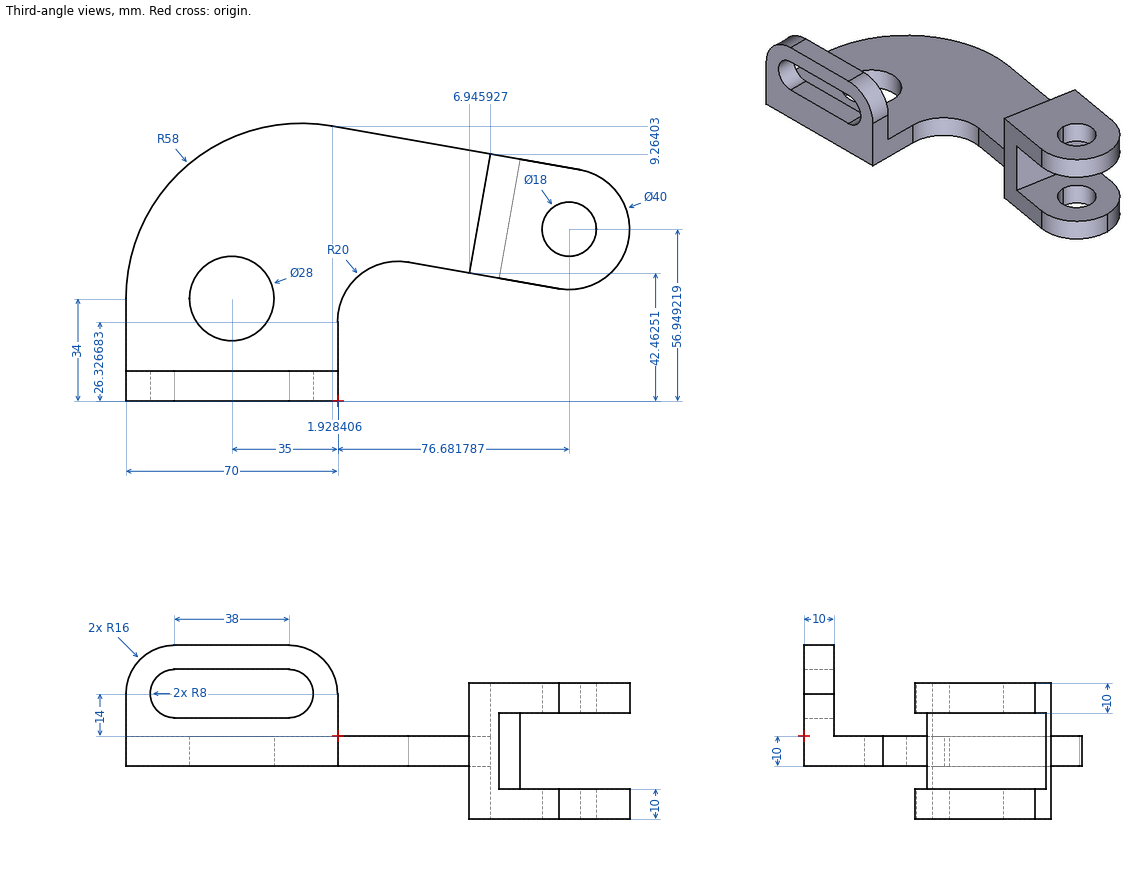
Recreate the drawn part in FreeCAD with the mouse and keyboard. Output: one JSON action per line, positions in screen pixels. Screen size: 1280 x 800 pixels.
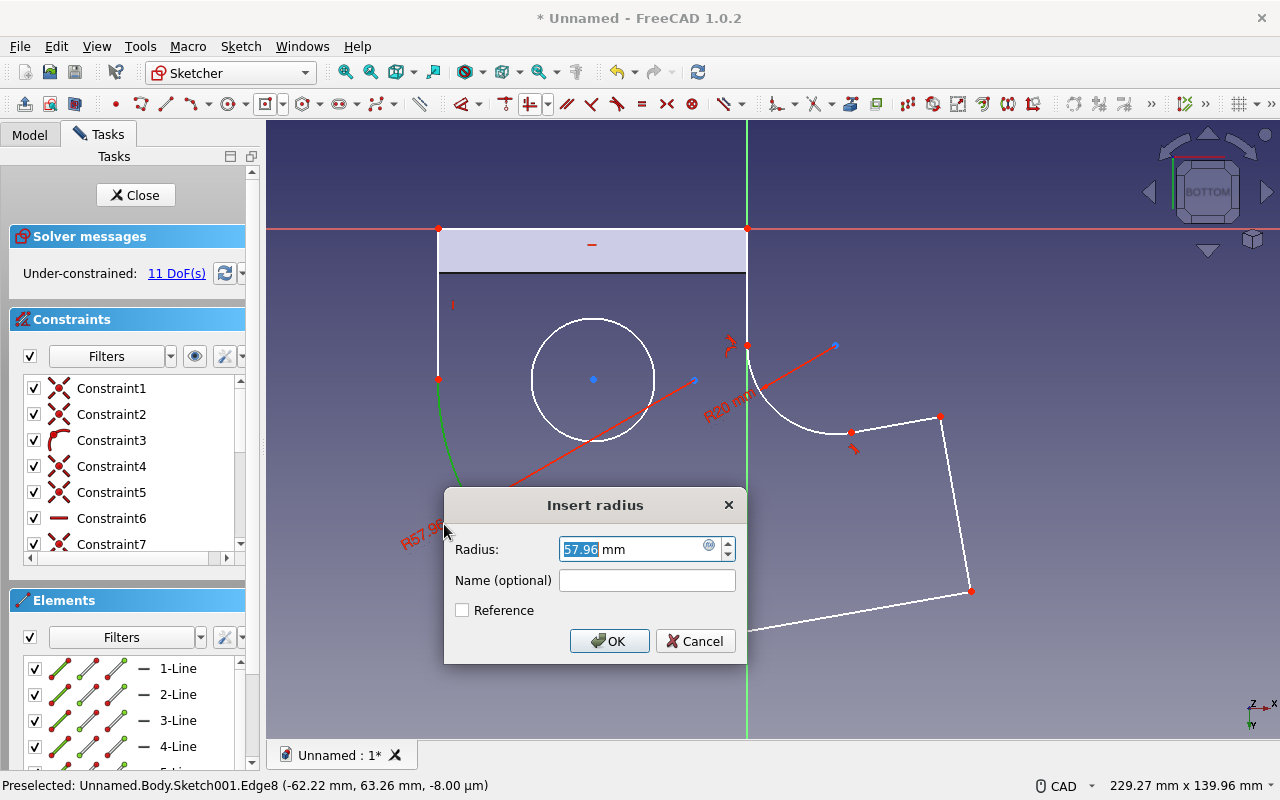
{"action": "type", "text": "58"}
{"action": "key", "text": "Return"}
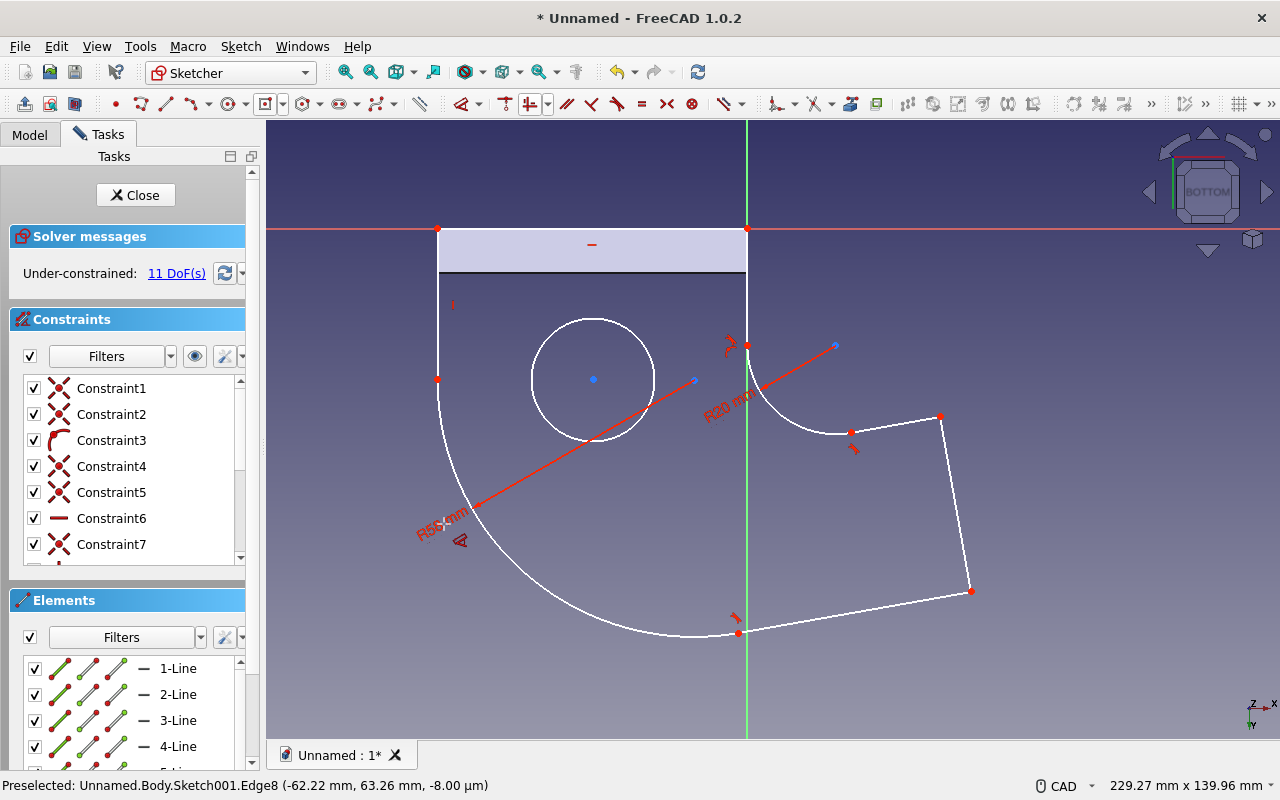
{"action": "left_click", "coordinate": [636, 336]}
{"action": "left_click", "coordinate": [658, 313]}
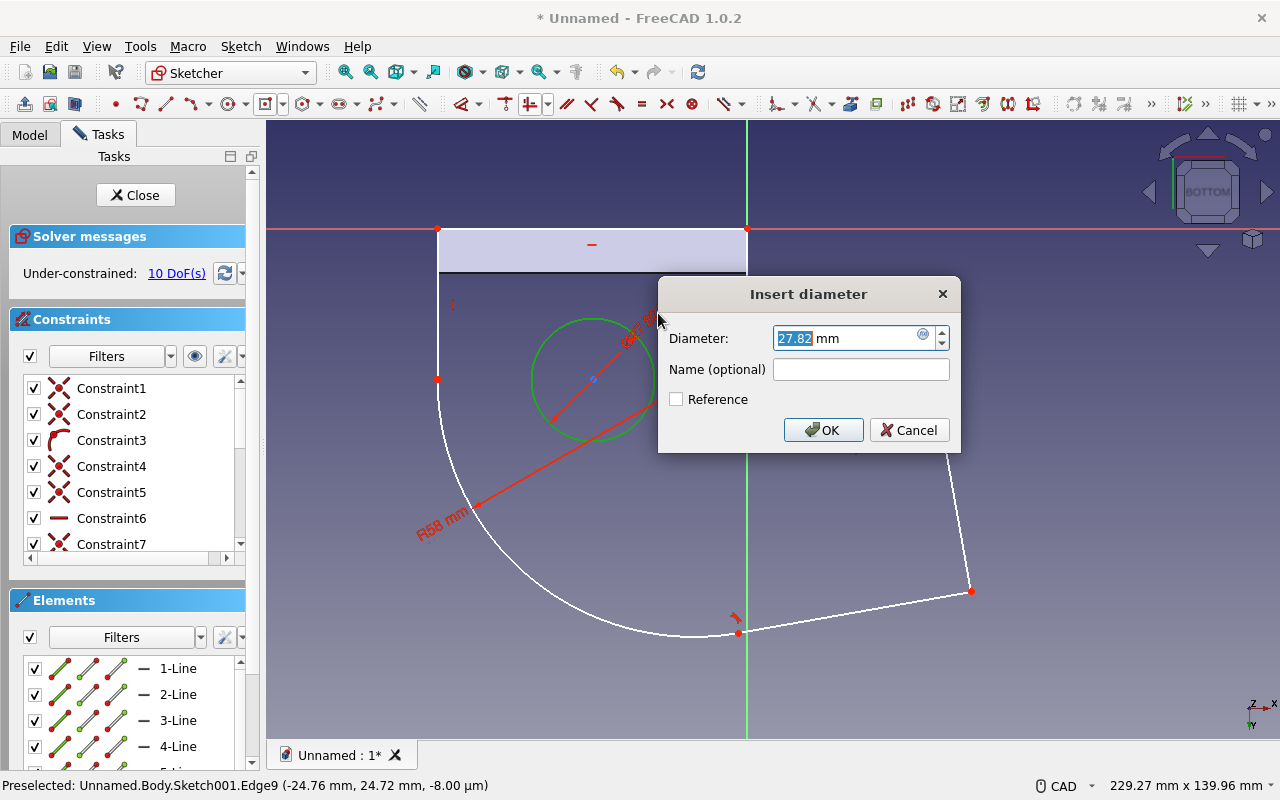
{"action": "type", "text": "28"}
{"action": "key", "text": "Return"}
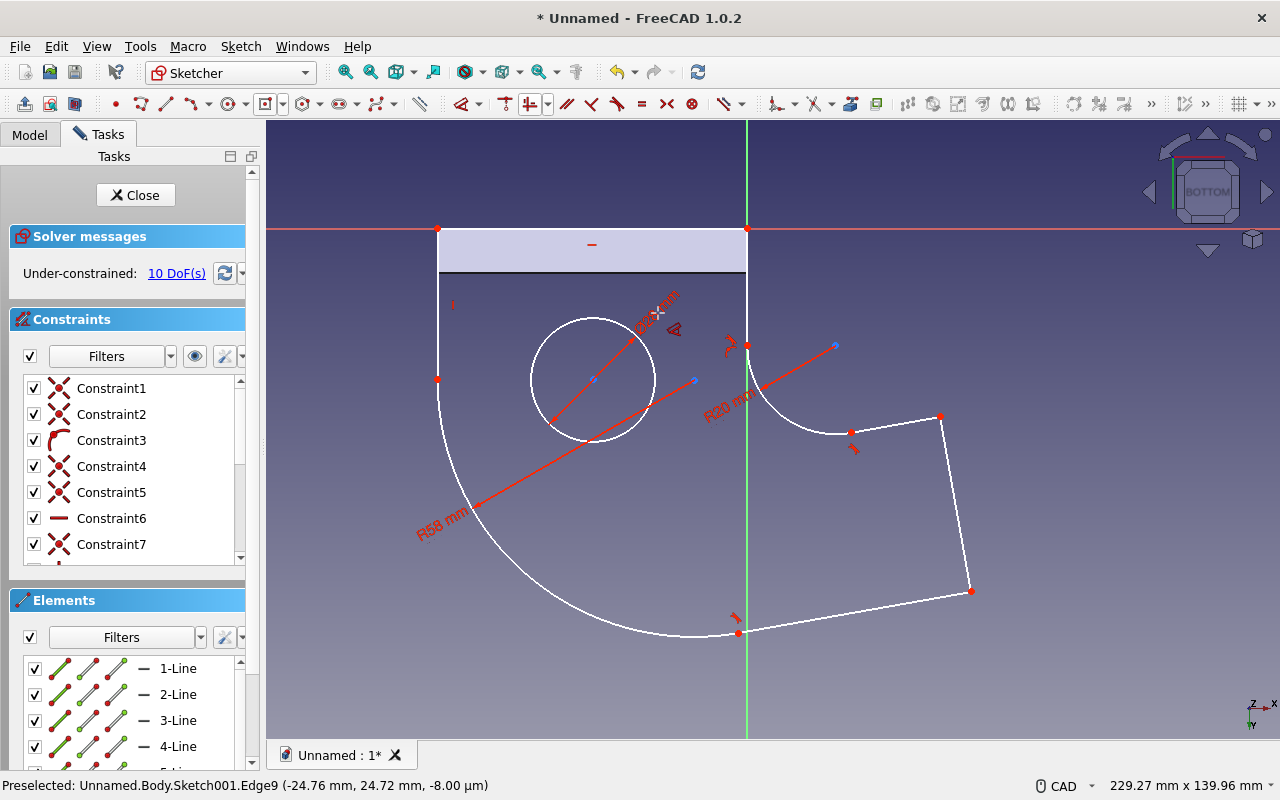
{"action": "left_click", "coordinate": [654, 229]}
{"action": "left_click", "coordinate": [593, 195]}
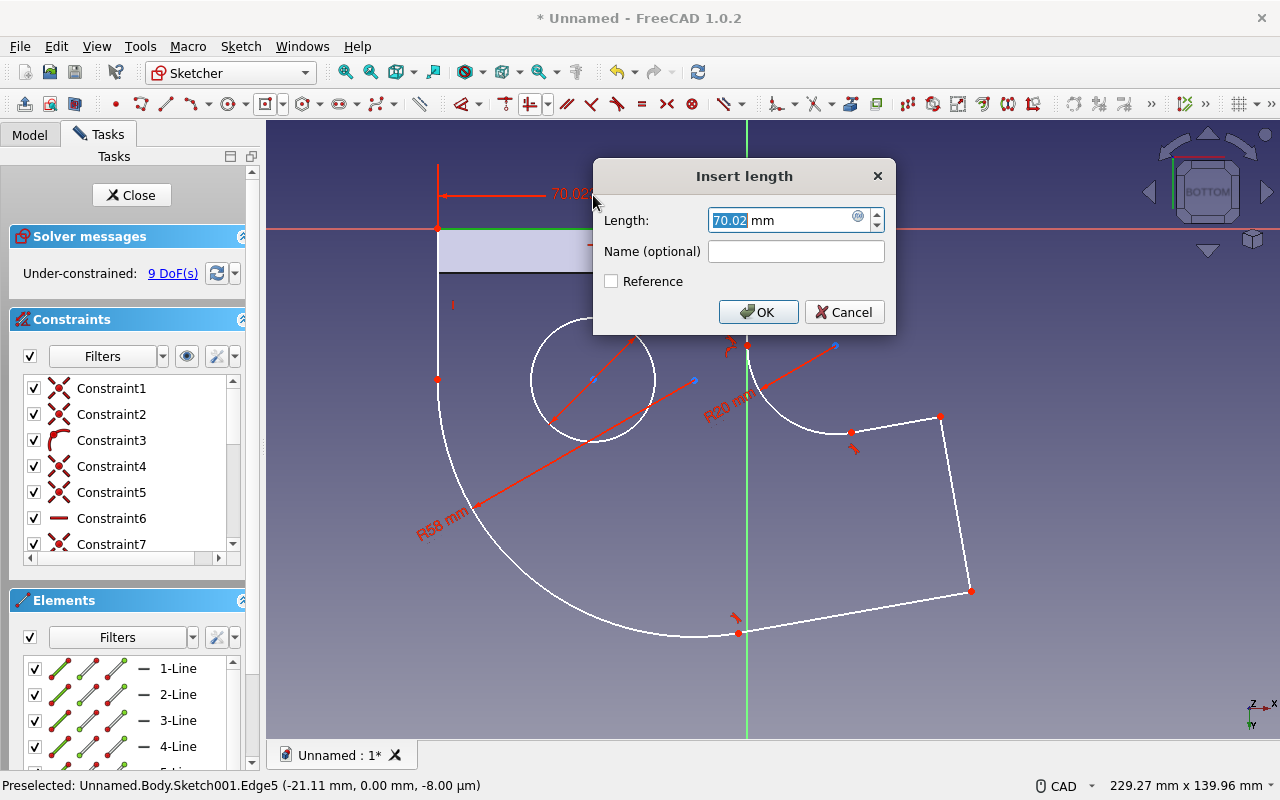
{"action": "type", "text": "70"}
{"action": "key", "text": "Return"}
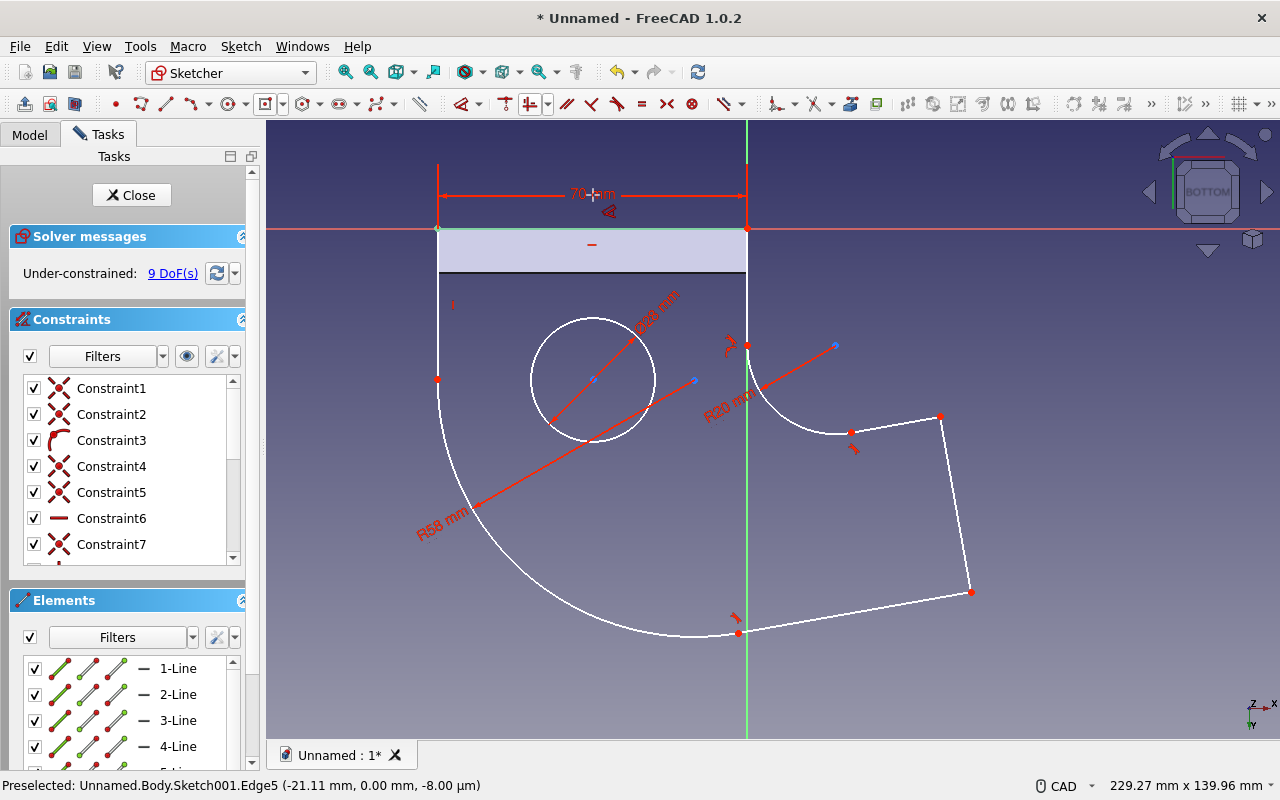
{"action": "left_click", "coordinate": [438, 274]}
{"action": "left_click", "coordinate": [404, 304]}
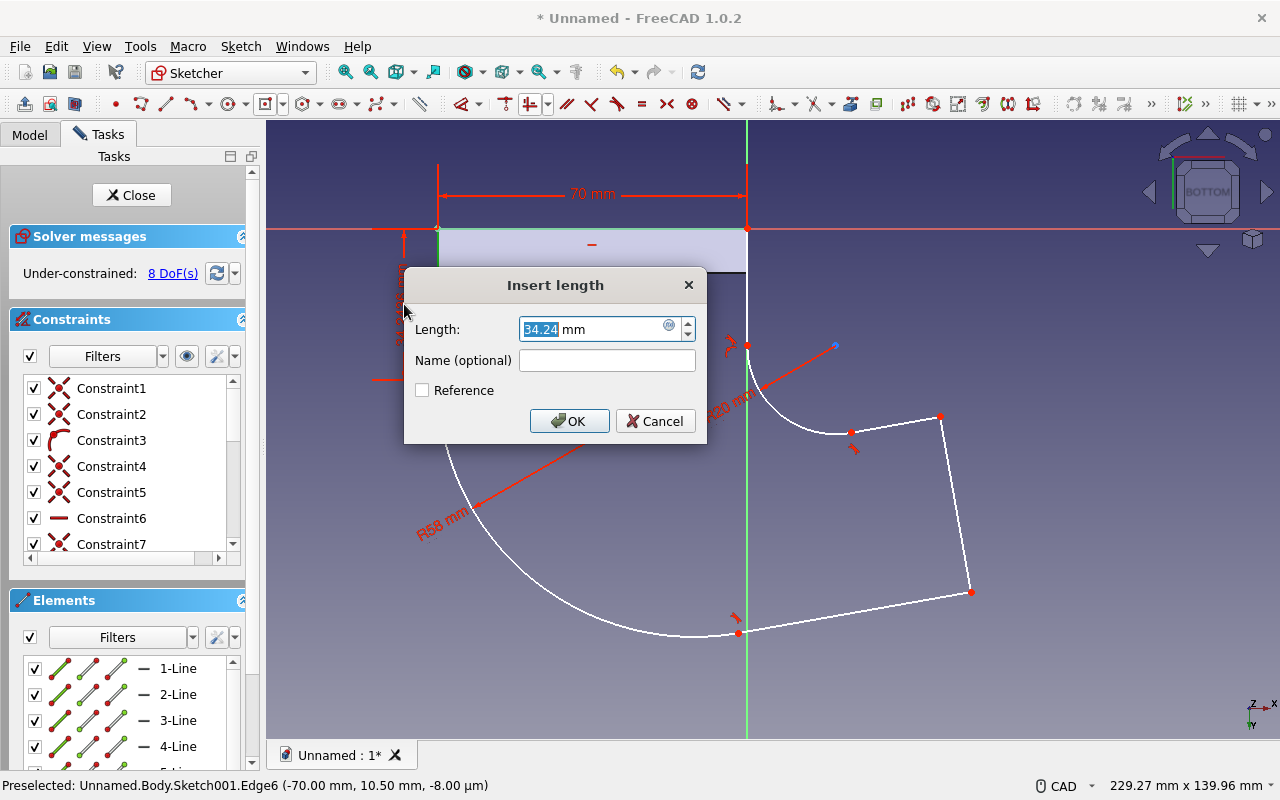
{"action": "type", "text": "34"}
{"action": "key", "text": "Return"}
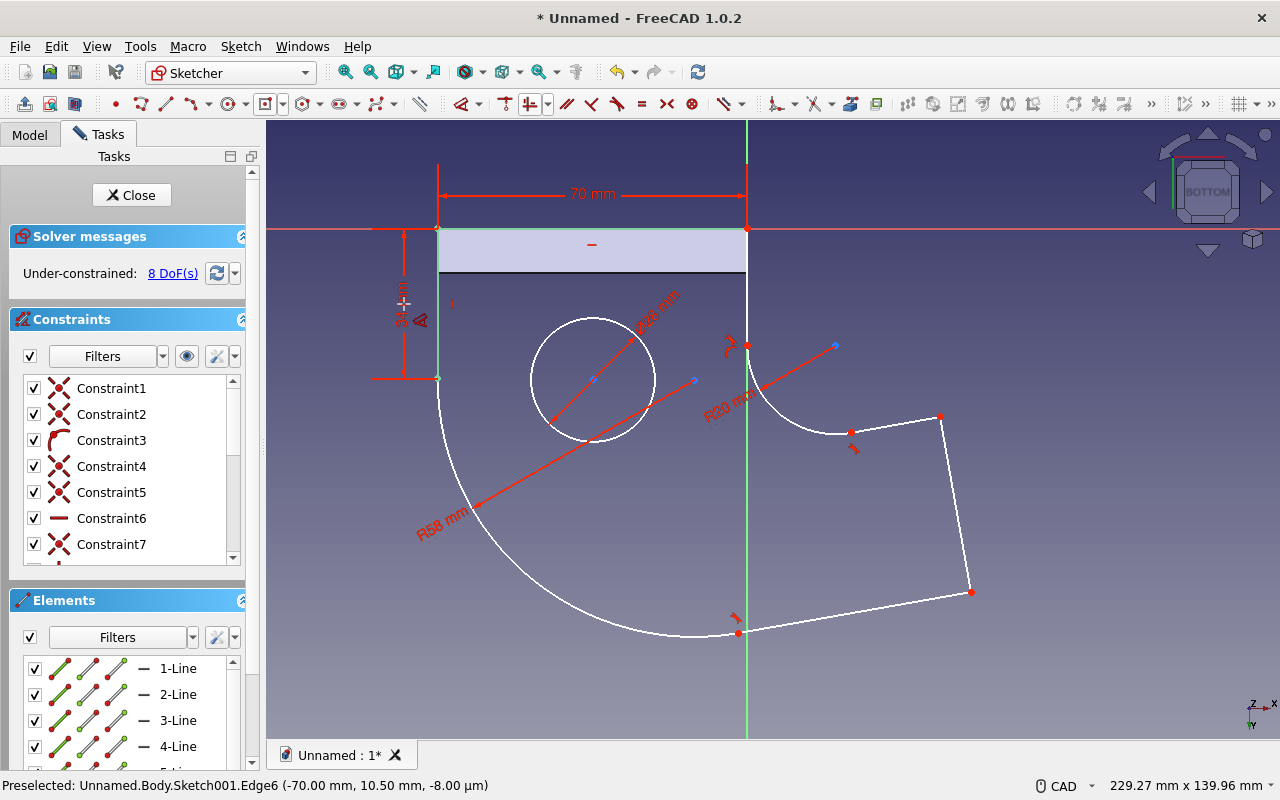
{"action": "left_click", "coordinate": [593, 380]}
{"action": "left_click", "coordinate": [670, 195]}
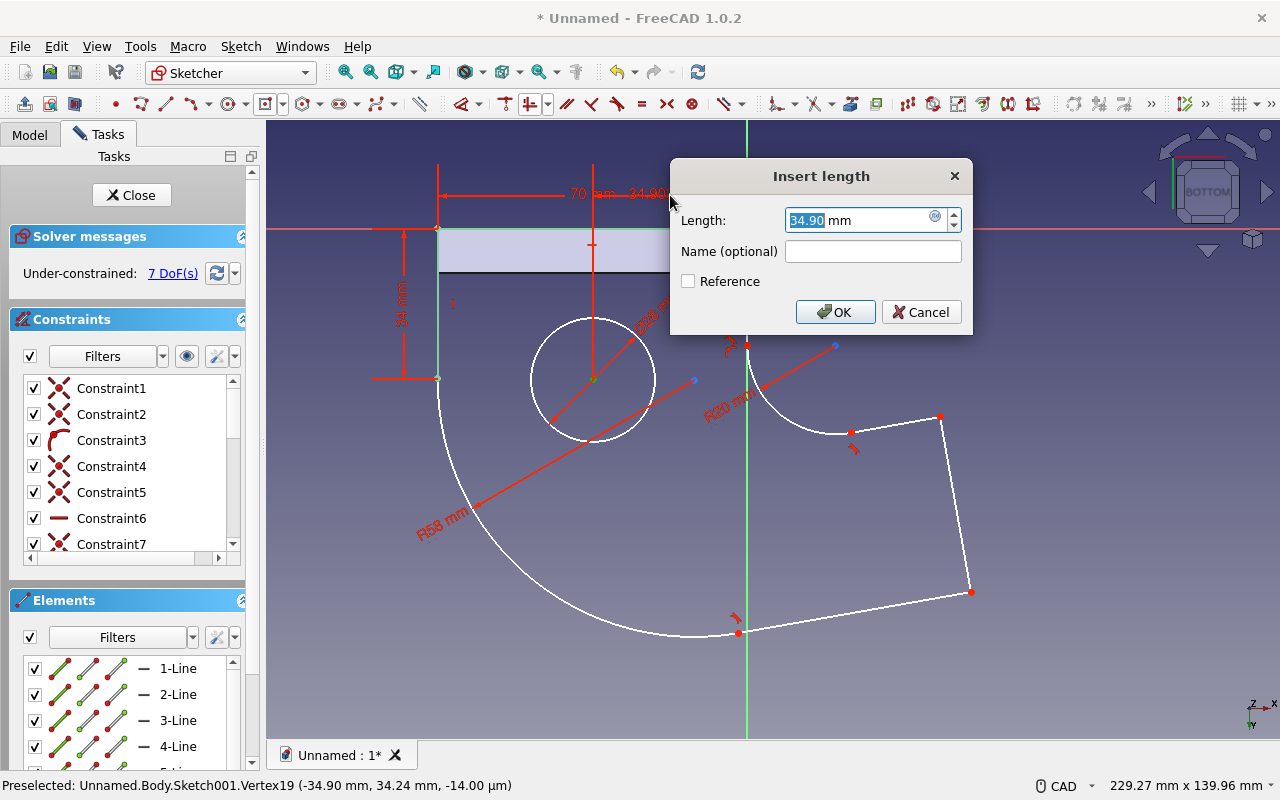
{"action": "type", "text": "35"}
{"action": "key", "text": "Return"}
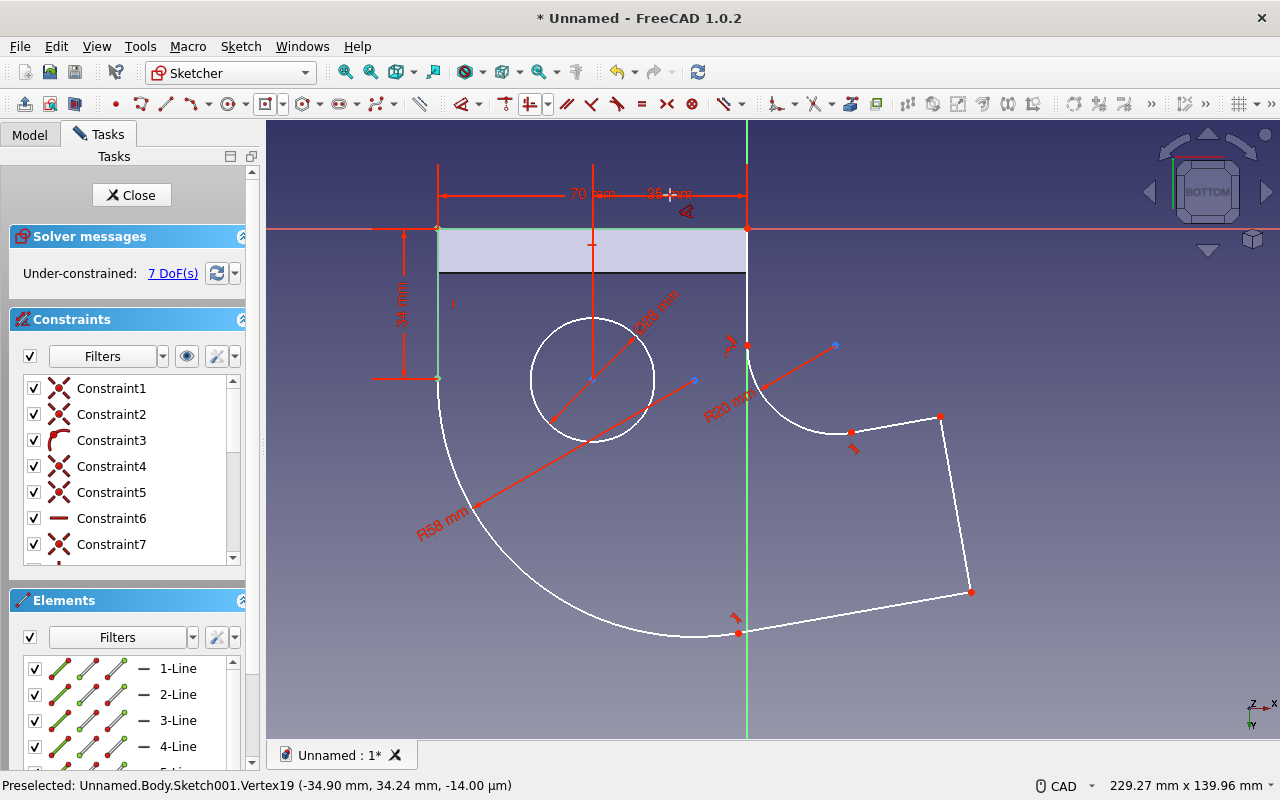
{"action": "left_click", "coordinate": [593, 380]}
{"action": "left_click", "coordinate": [559, 304]}